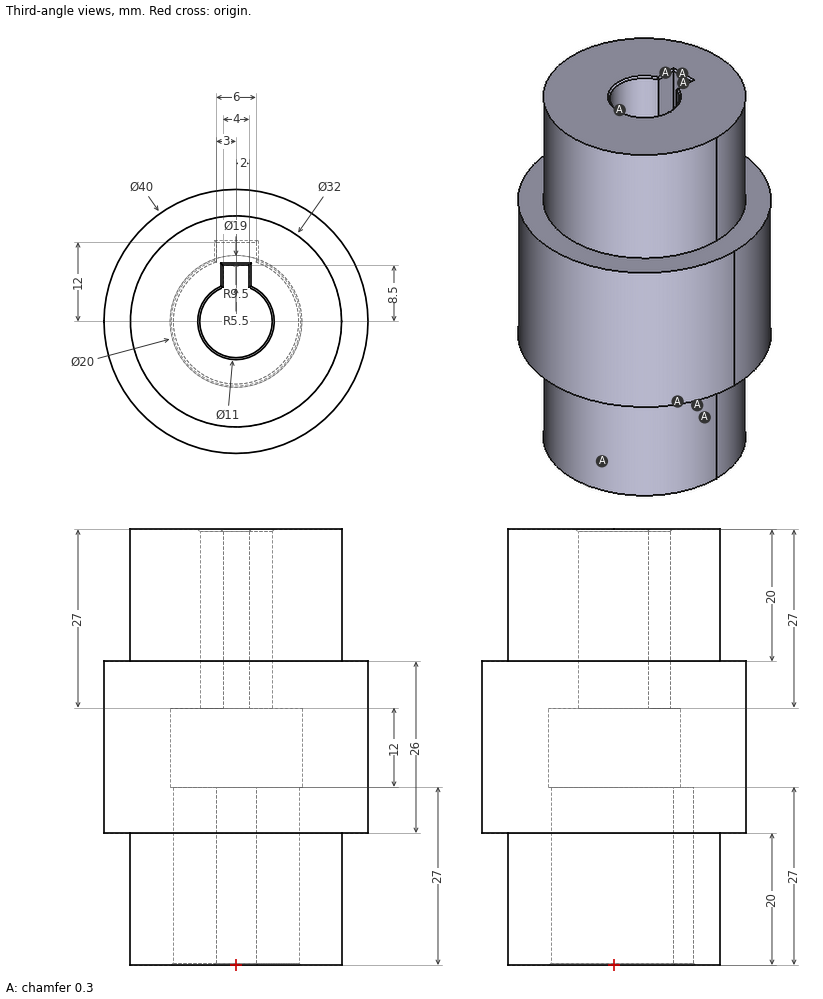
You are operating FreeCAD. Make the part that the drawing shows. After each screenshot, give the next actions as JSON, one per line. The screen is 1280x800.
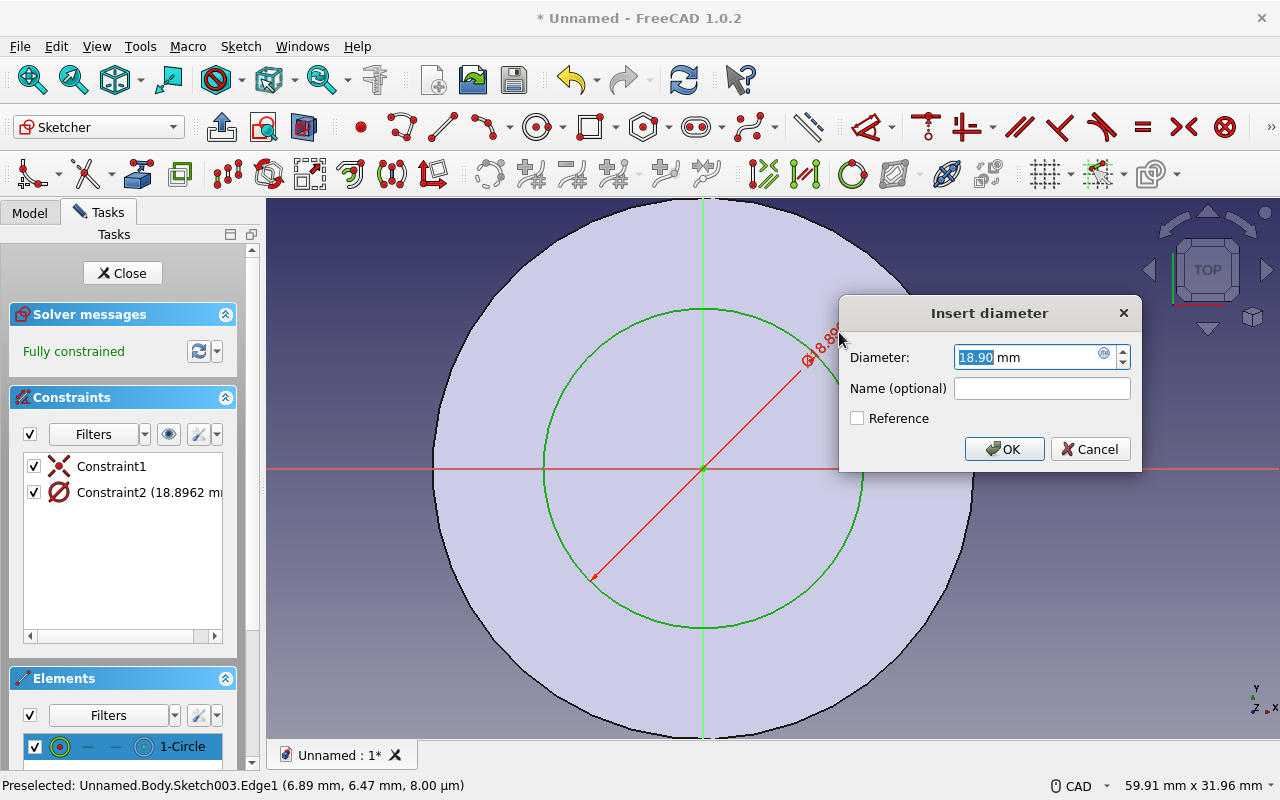
{"action": "type", "text": "19"}
{"action": "key", "text": "Return"}
{"action": "key", "text": "Escape"}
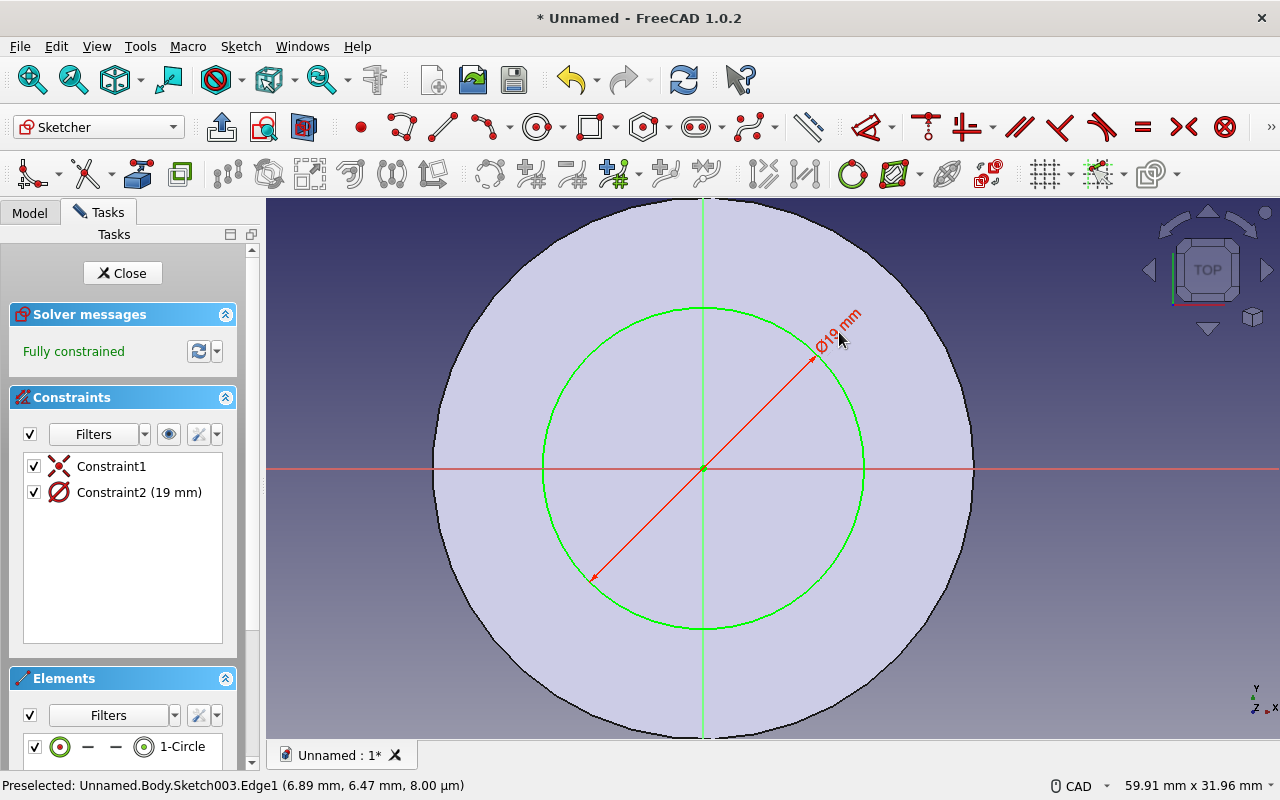
{"action": "left_click", "coordinate": [123, 273]}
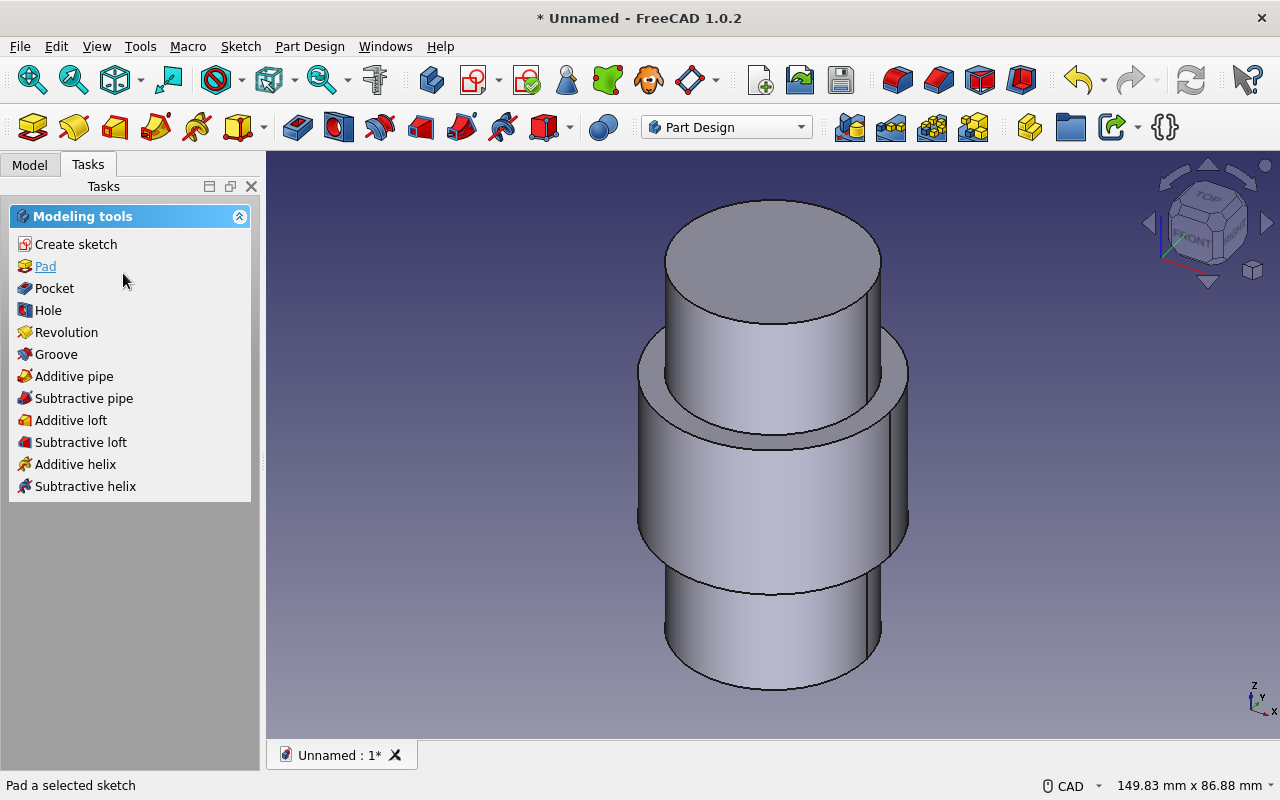
{"action": "left_click", "coordinate": [298, 128]}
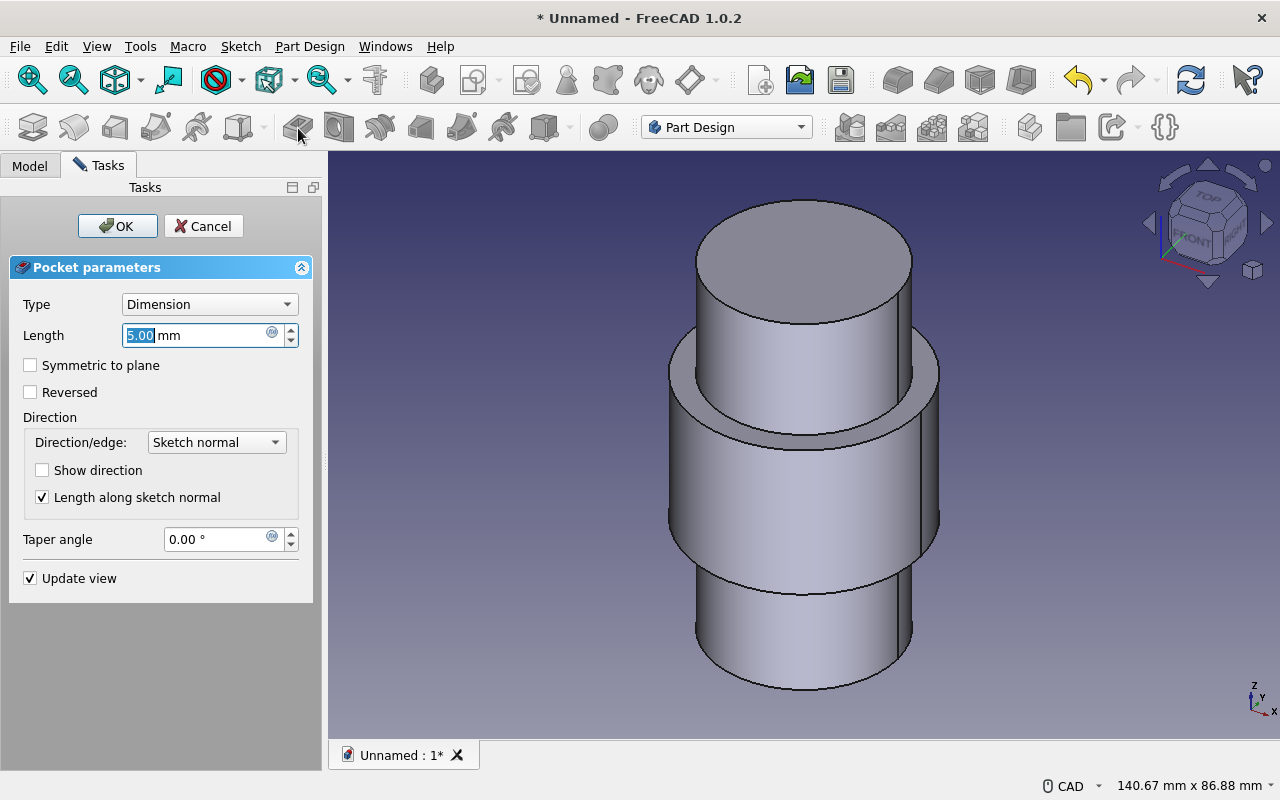
{"action": "type", "text": "27"}
{"action": "key", "text": "Tab"}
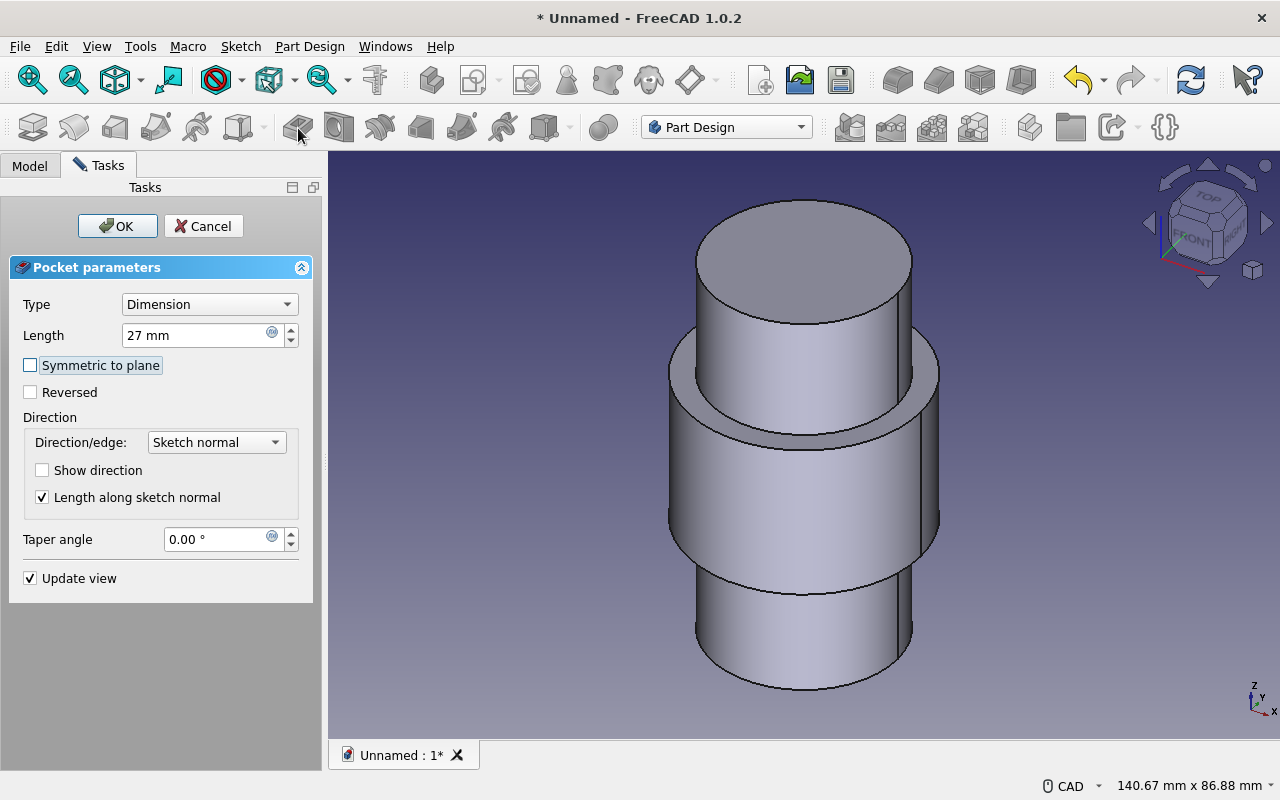
{"action": "left_click", "coordinate": [31, 392]}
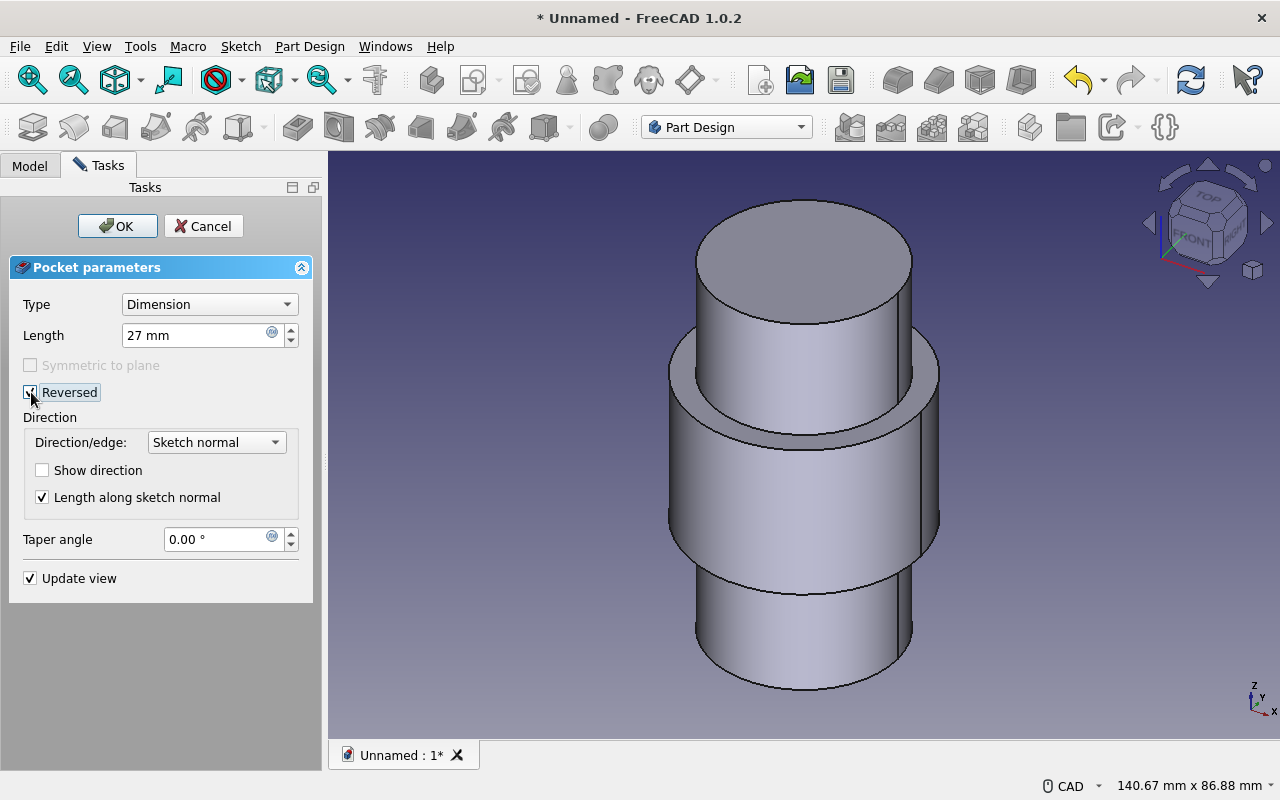
{"action": "left_click", "coordinate": [118, 226]}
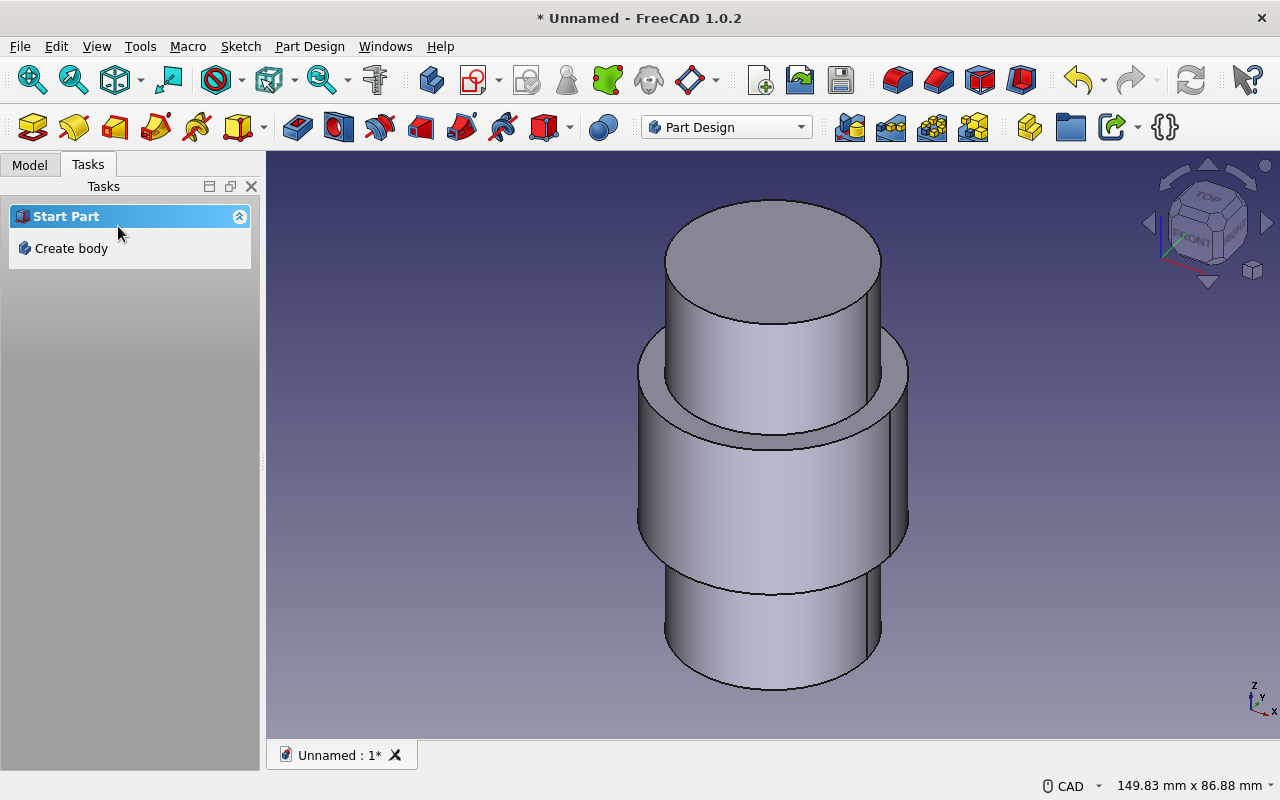
{"action": "left_click", "coordinate": [773, 261]}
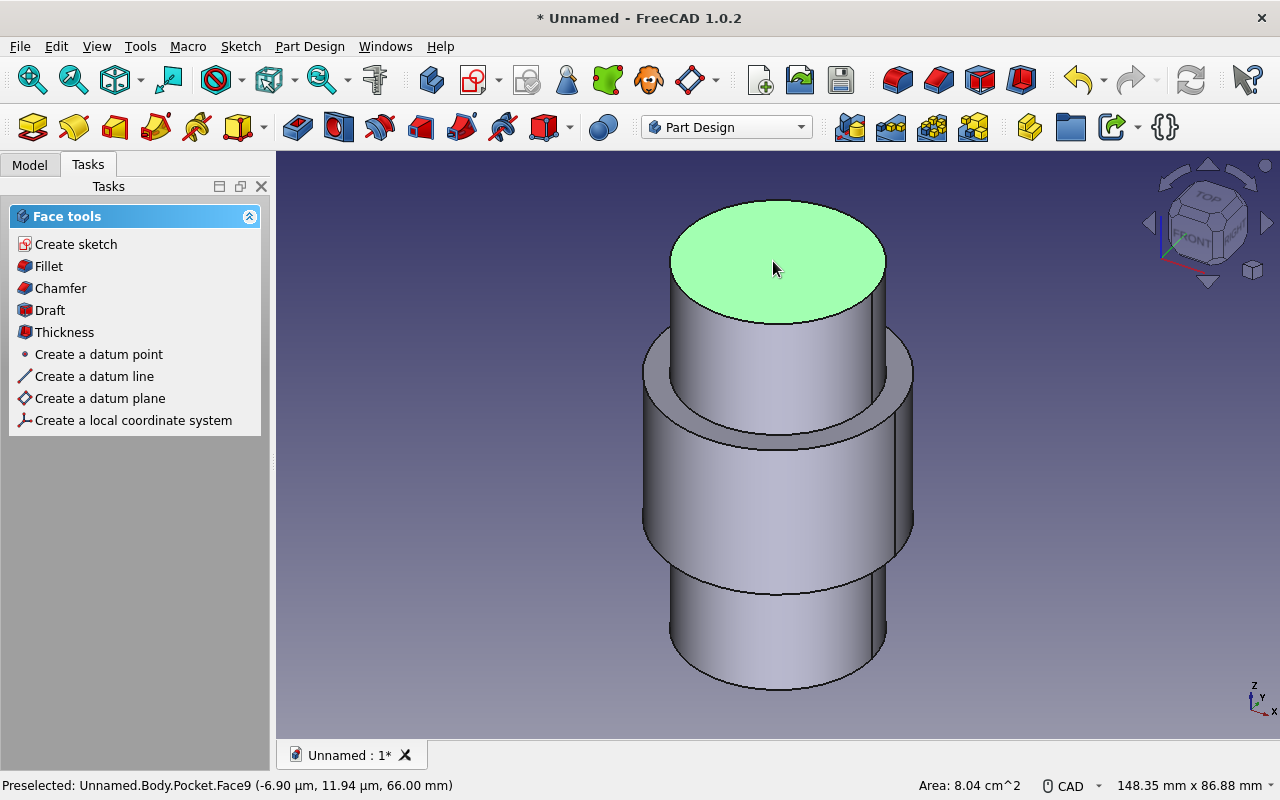
{"action": "left_click", "coordinate": [472, 80]}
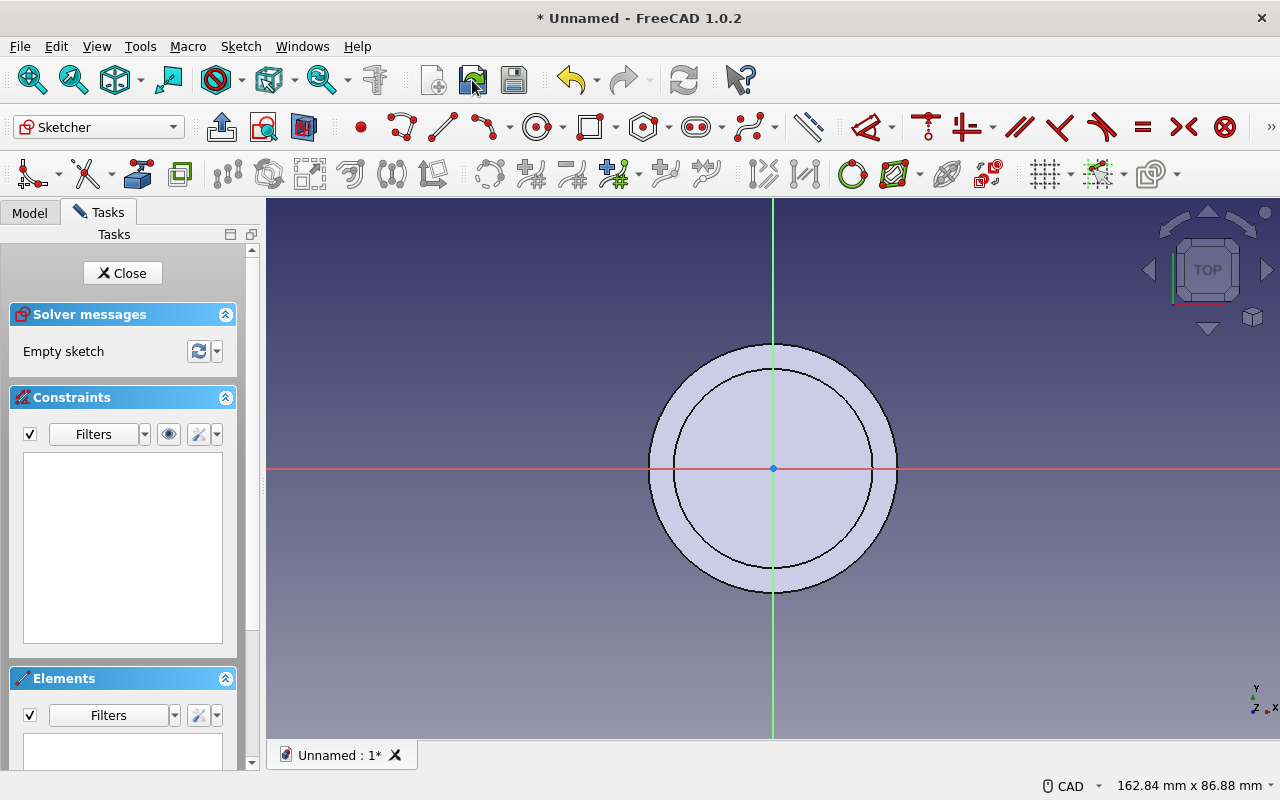
{"action": "scroll", "coordinate": [790, 469], "scroll_direction": "up", "scroll_amount": 8}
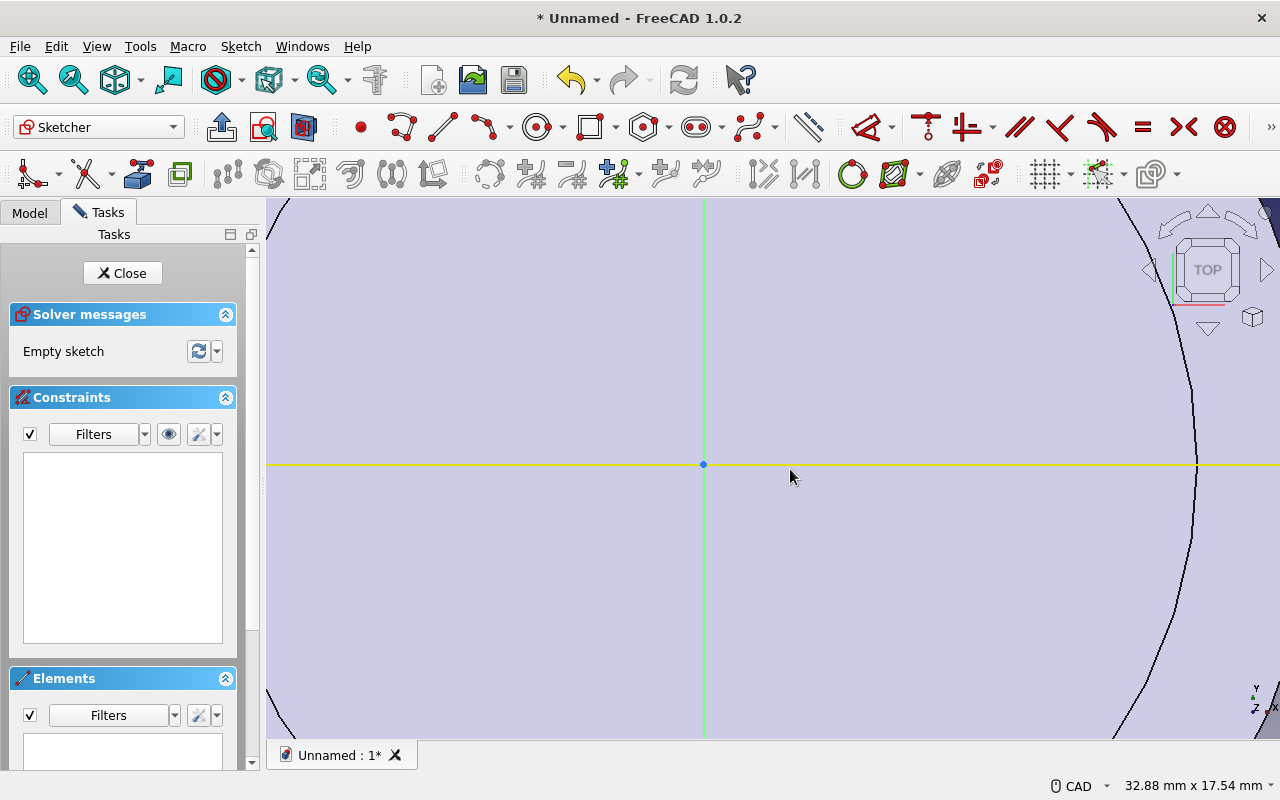
{"action": "left_click", "coordinate": [536, 128]}